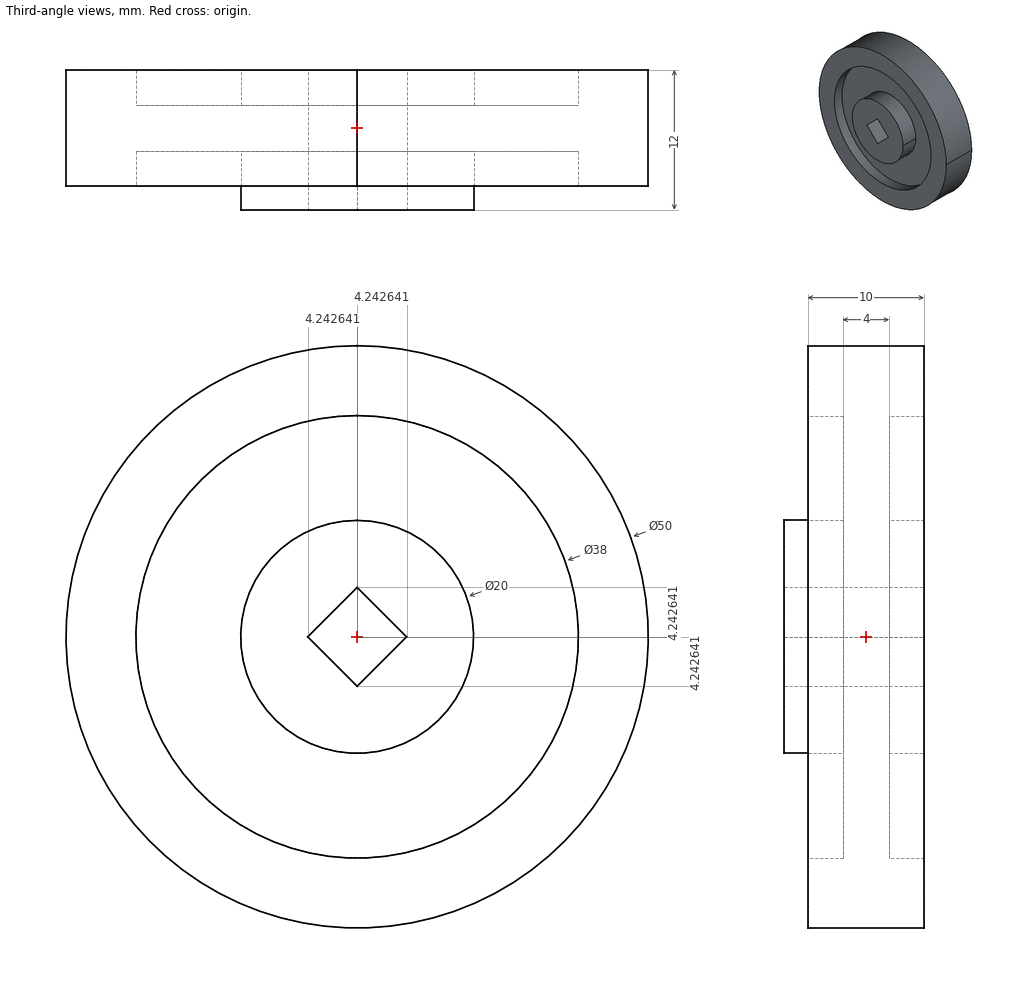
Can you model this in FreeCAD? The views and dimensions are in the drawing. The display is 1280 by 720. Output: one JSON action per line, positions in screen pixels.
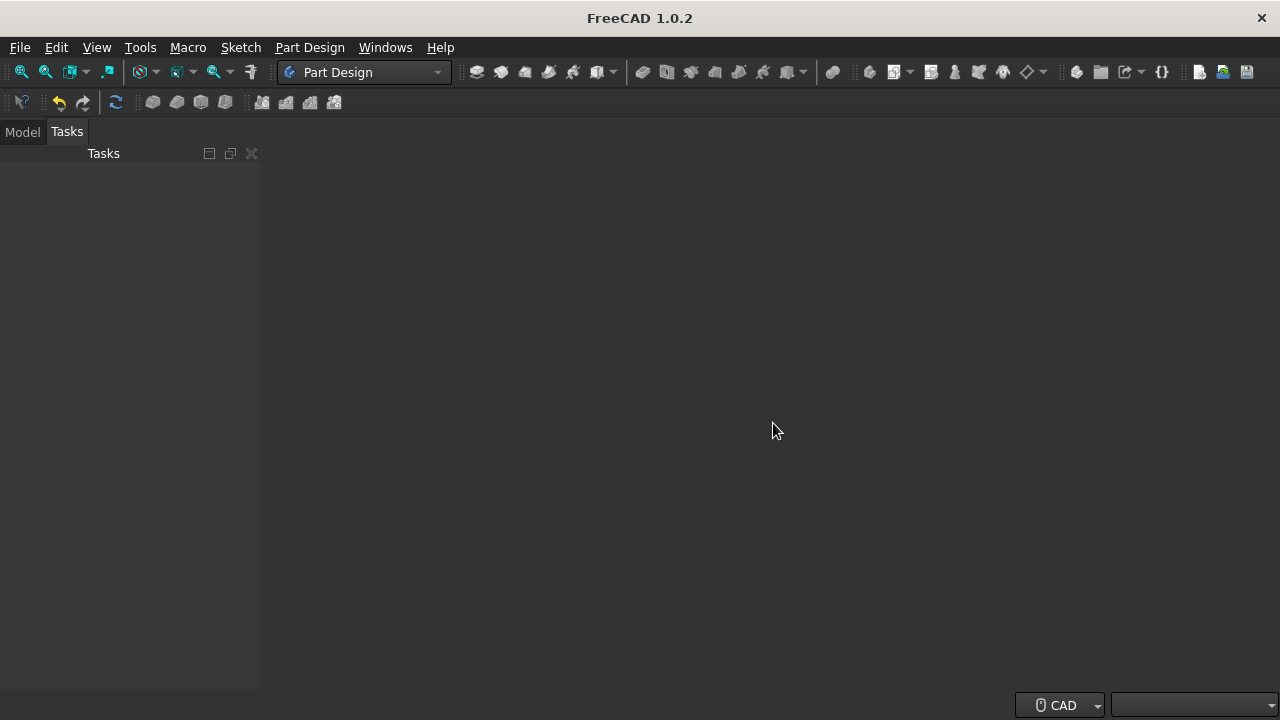
{"action": "left_click", "coordinate": [1200, 72]}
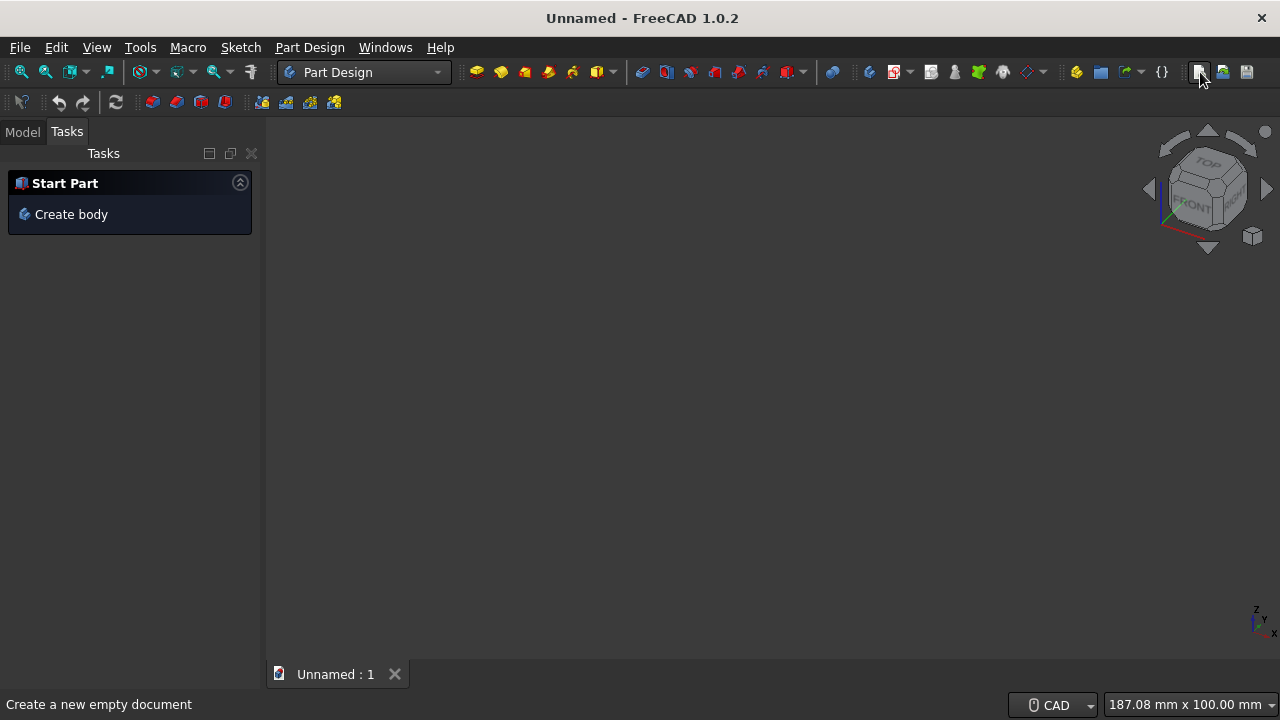
{"action": "left_click", "coordinate": [894, 72]}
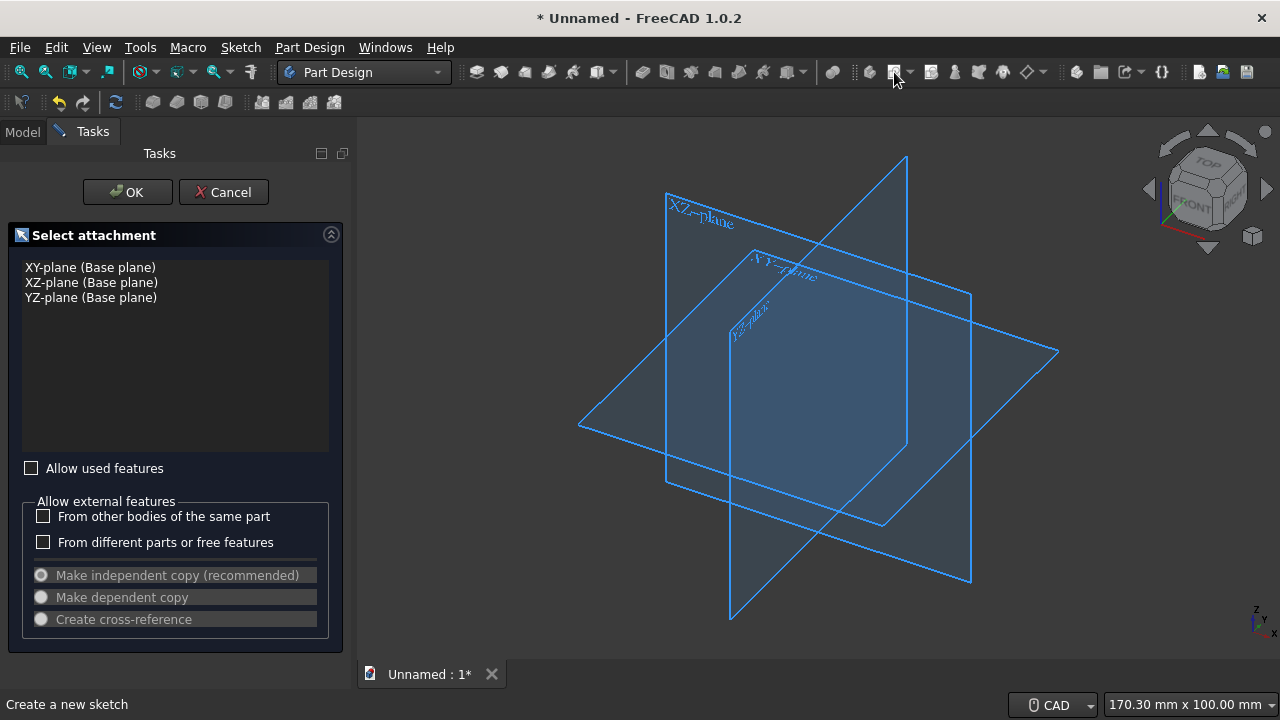
{"action": "left_click", "coordinate": [82, 282]}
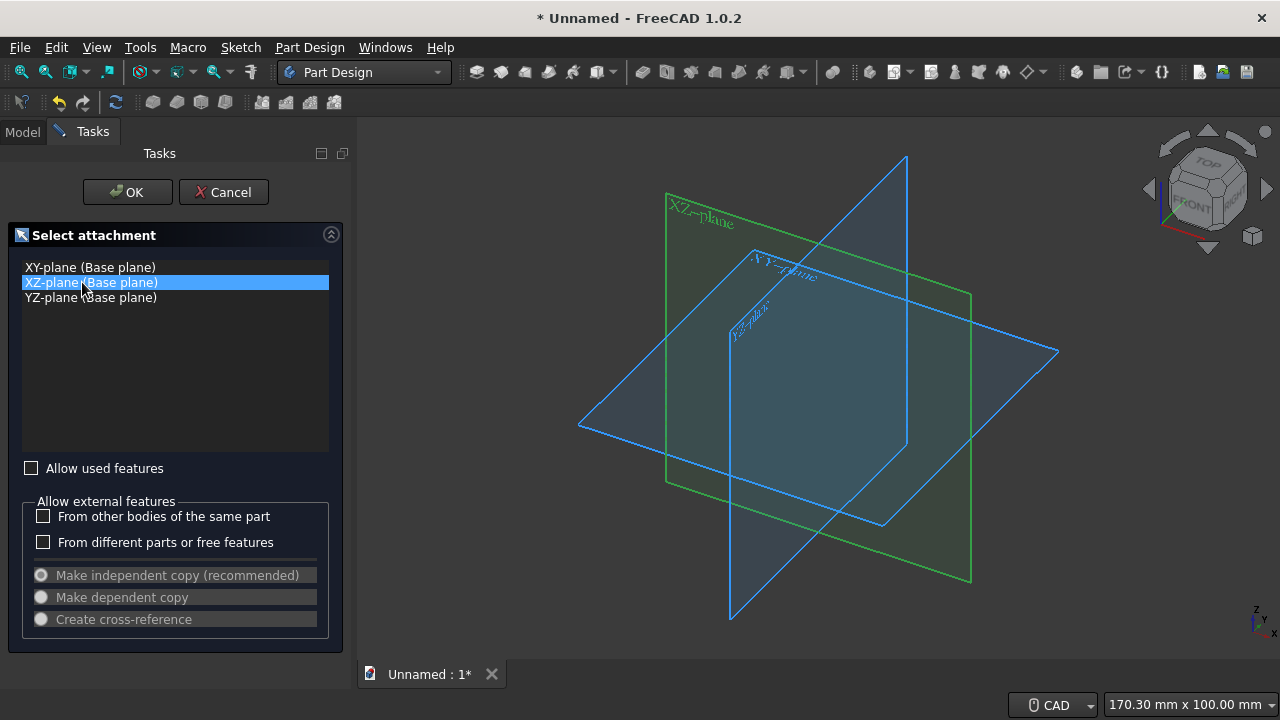
{"action": "left_click", "coordinate": [128, 192]}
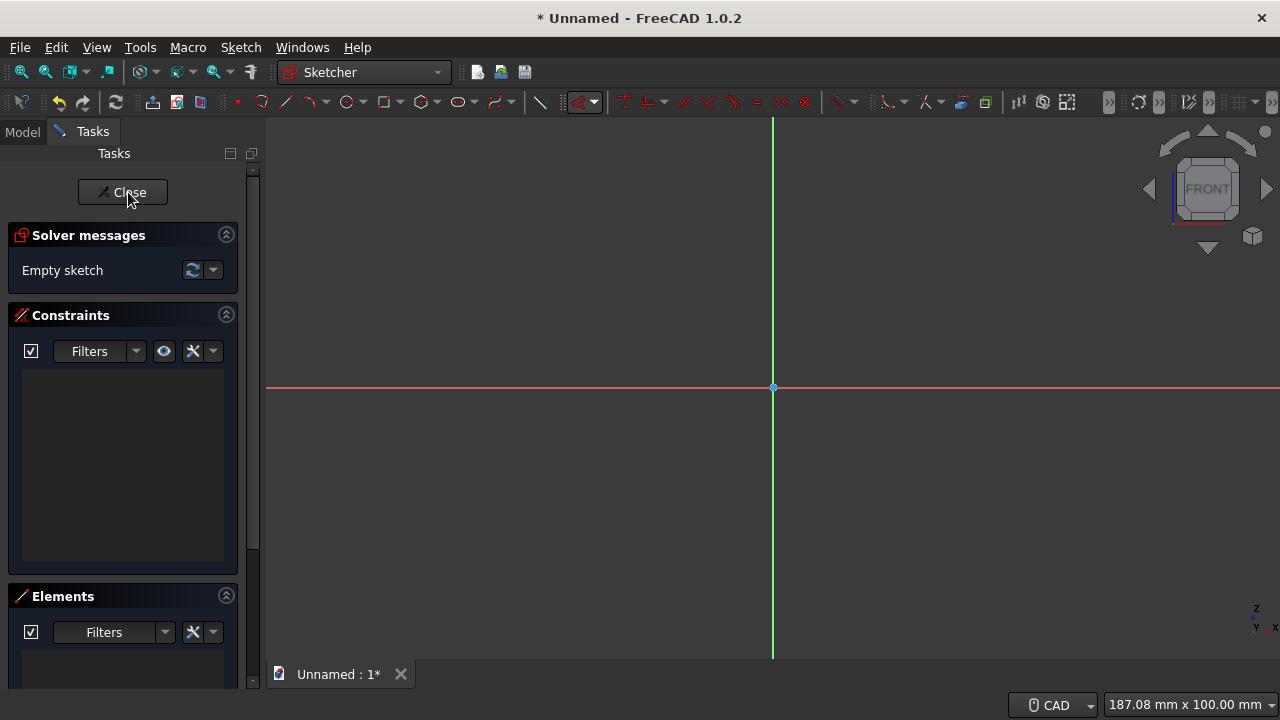
{"action": "left_click", "coordinate": [348, 102]}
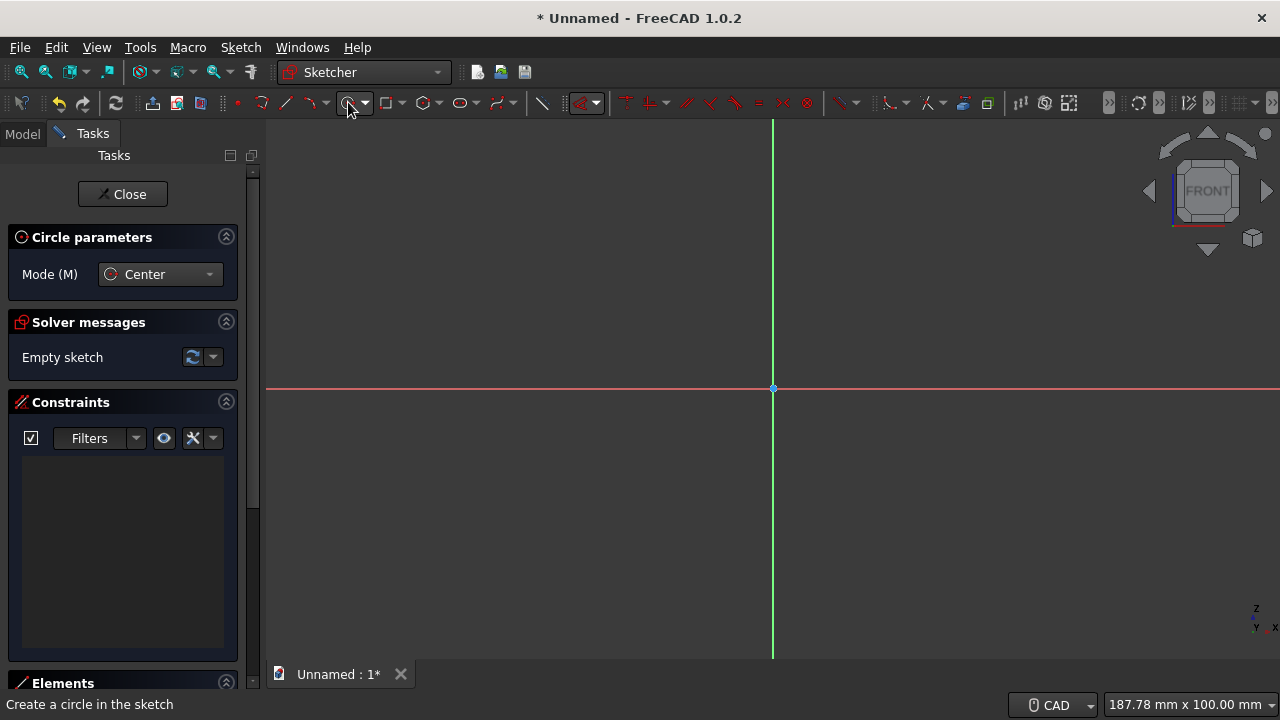
{"action": "left_click", "coordinate": [773, 389]}
{"action": "left_click", "coordinate": [868, 294]}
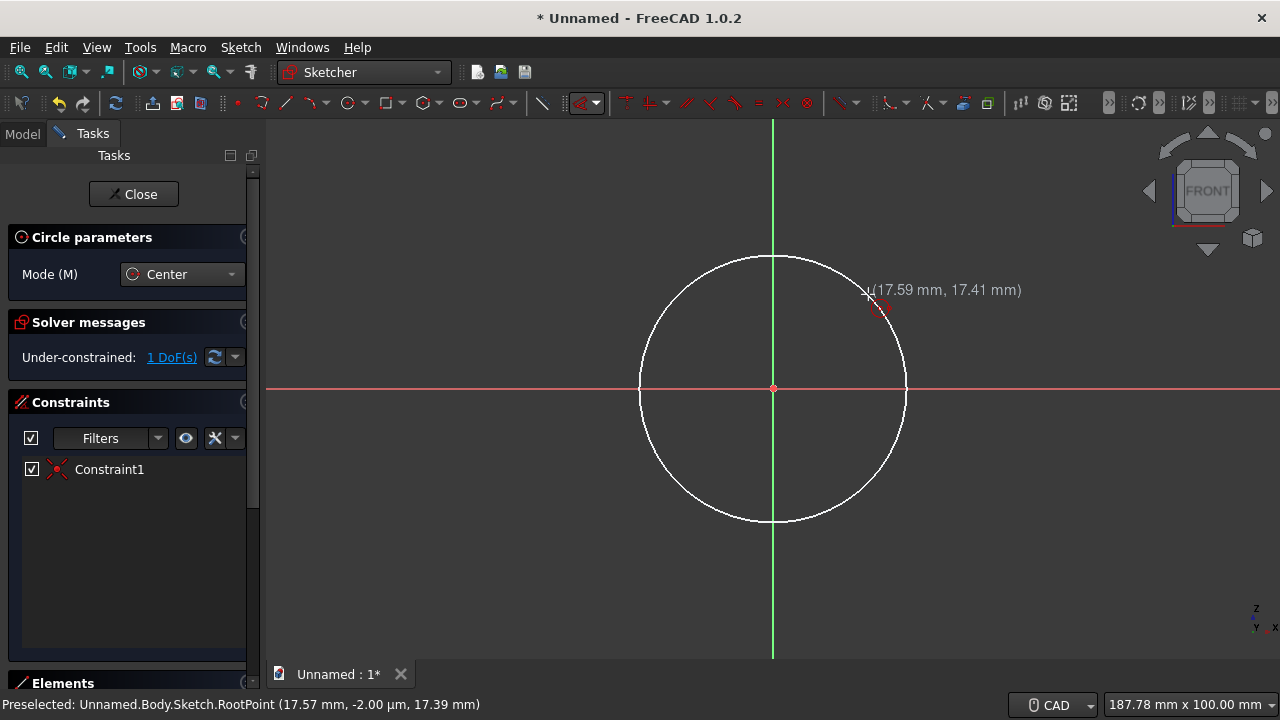
{"action": "left_click", "coordinate": [773, 389]}
{"action": "left_click", "coordinate": [846, 316]}
{"action": "key", "text": "Escape"}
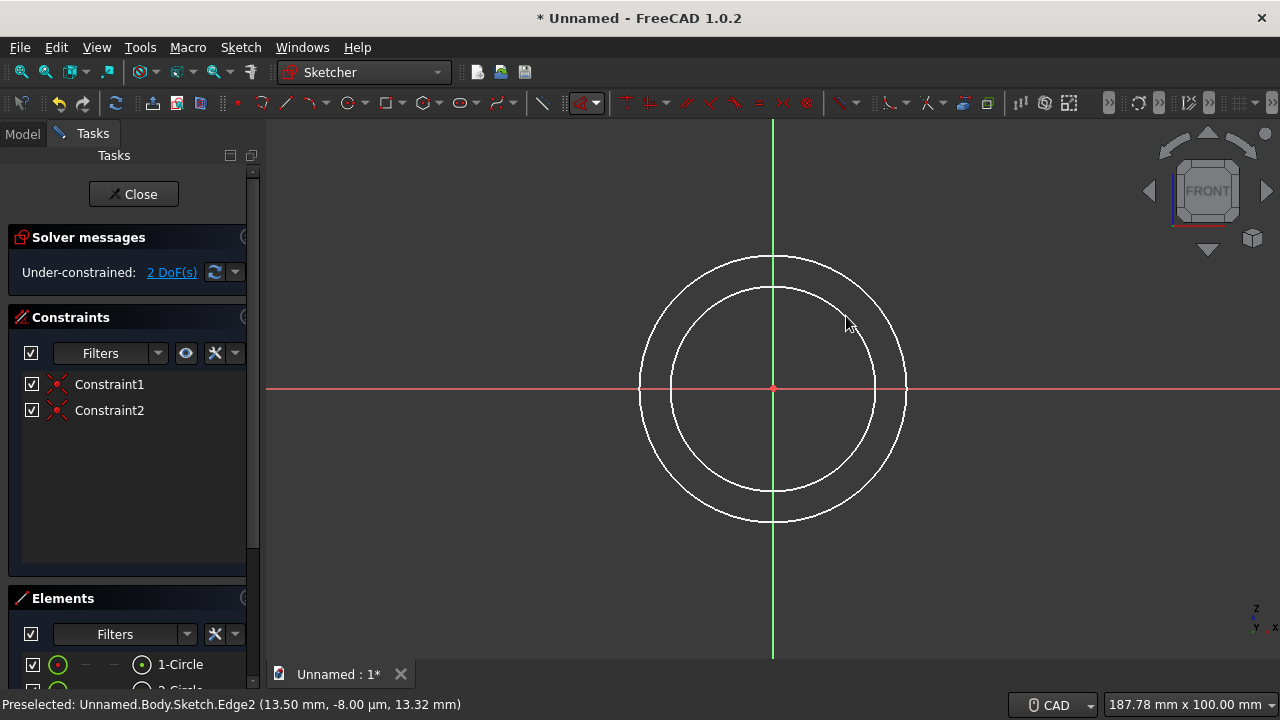
{"action": "left_click", "coordinate": [580, 104]}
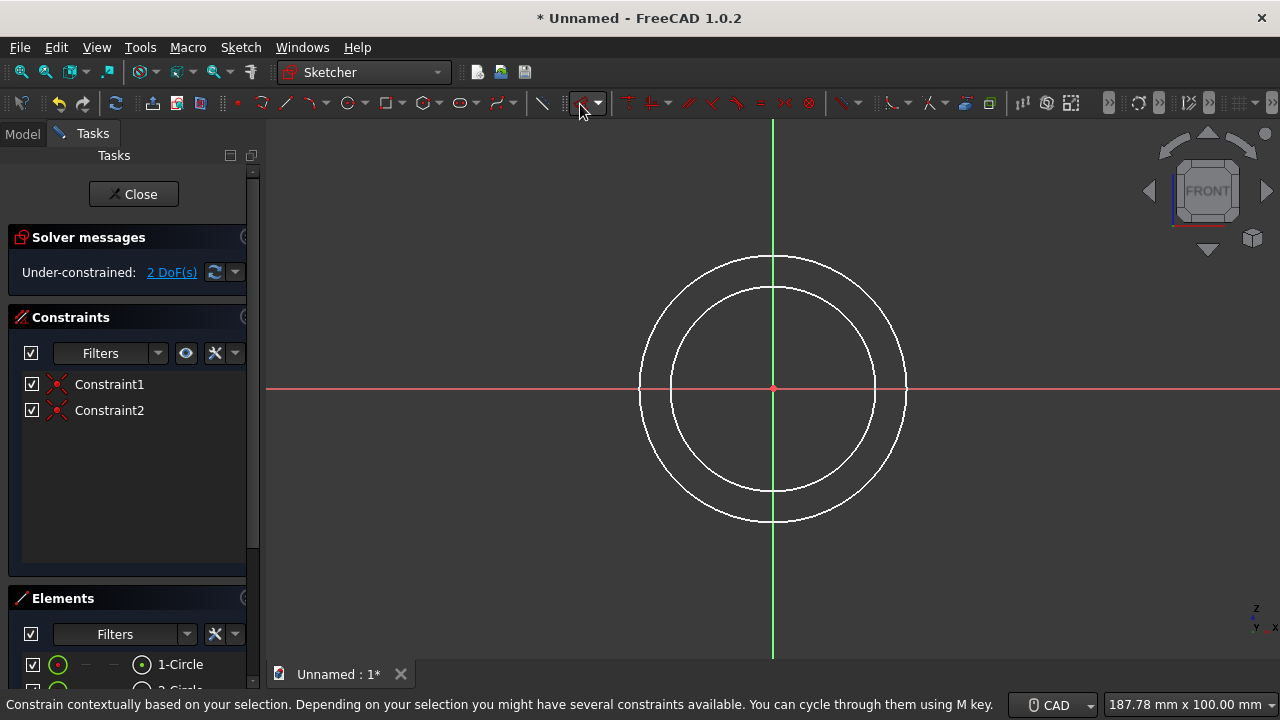
{"action": "left_click", "coordinate": [867, 294]}
{"action": "left_click", "coordinate": [890, 271]}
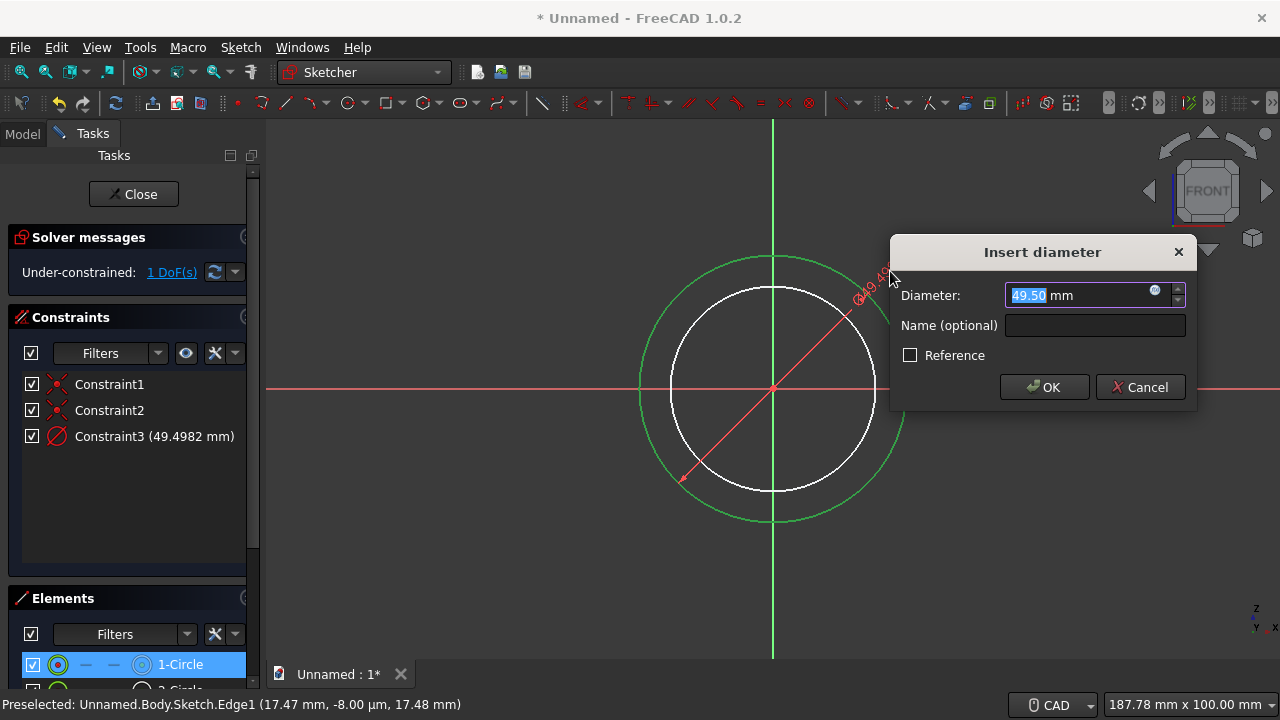
{"action": "type", "text": "50"}
{"action": "key", "text": "Return"}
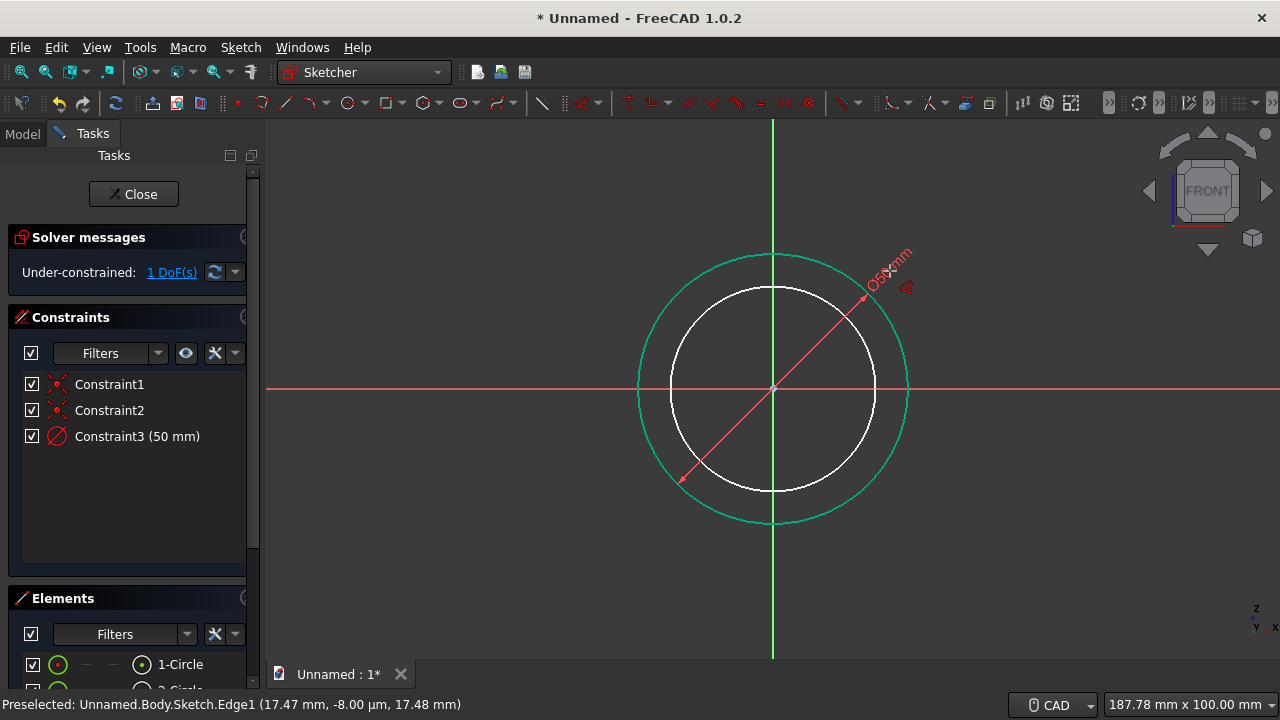
{"action": "left_click", "coordinate": [845, 316]}
{"action": "left_click", "coordinate": [924, 344]}